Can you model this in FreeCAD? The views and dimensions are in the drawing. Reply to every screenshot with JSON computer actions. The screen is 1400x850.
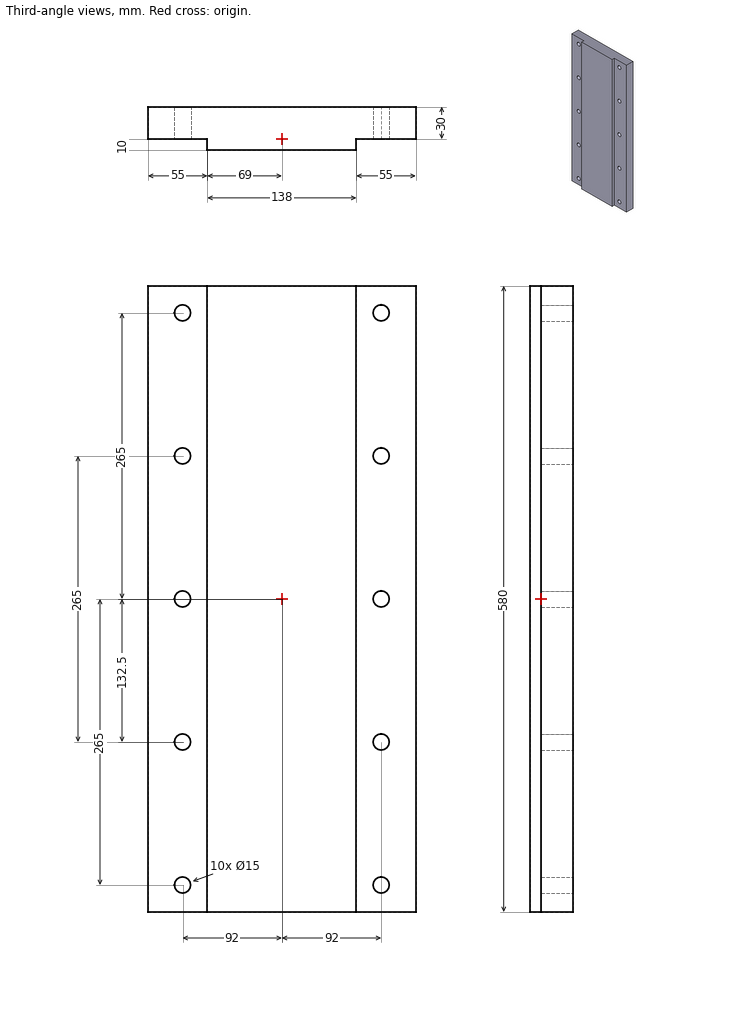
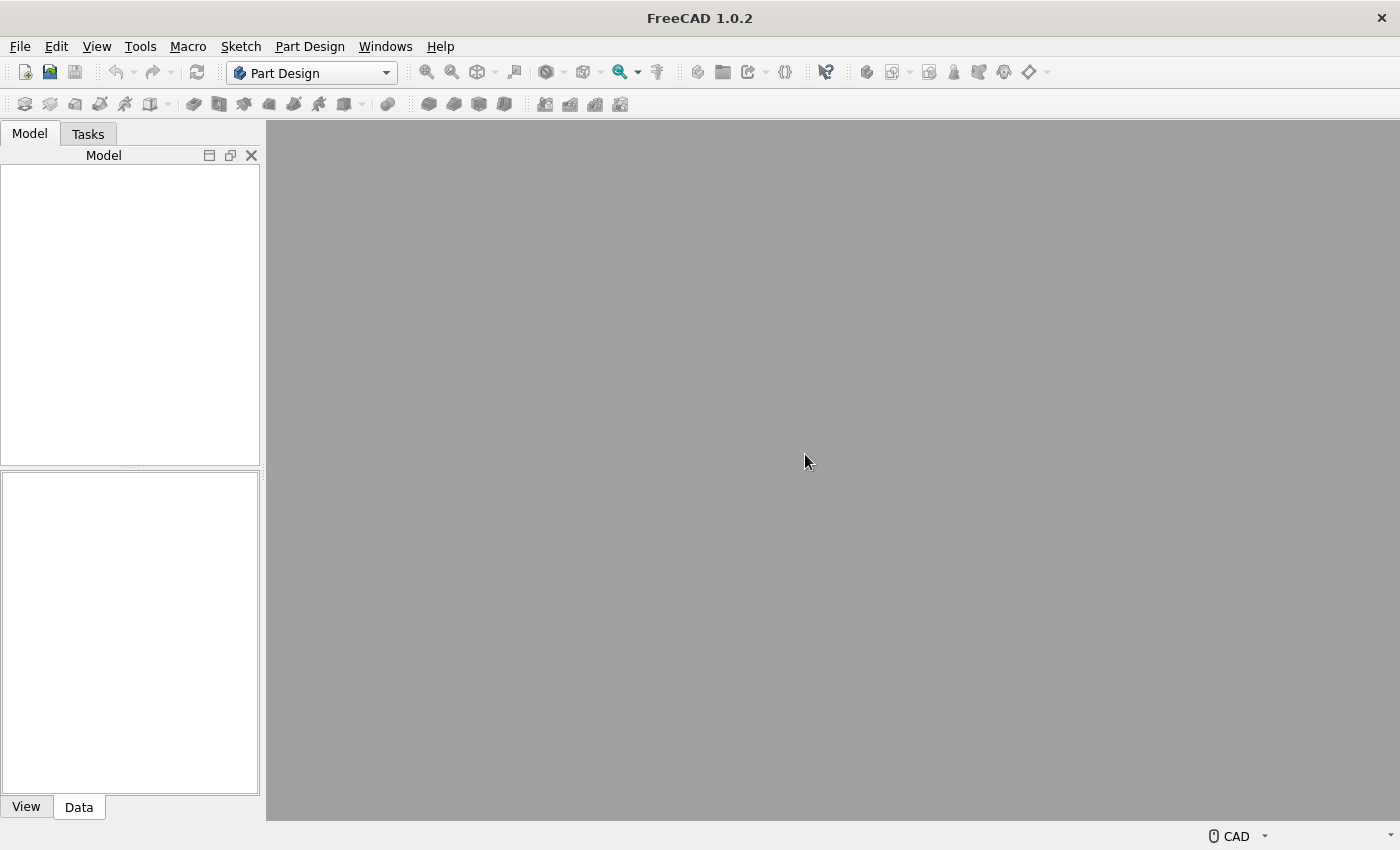
{"action": "left_click", "coordinate": [25, 72]}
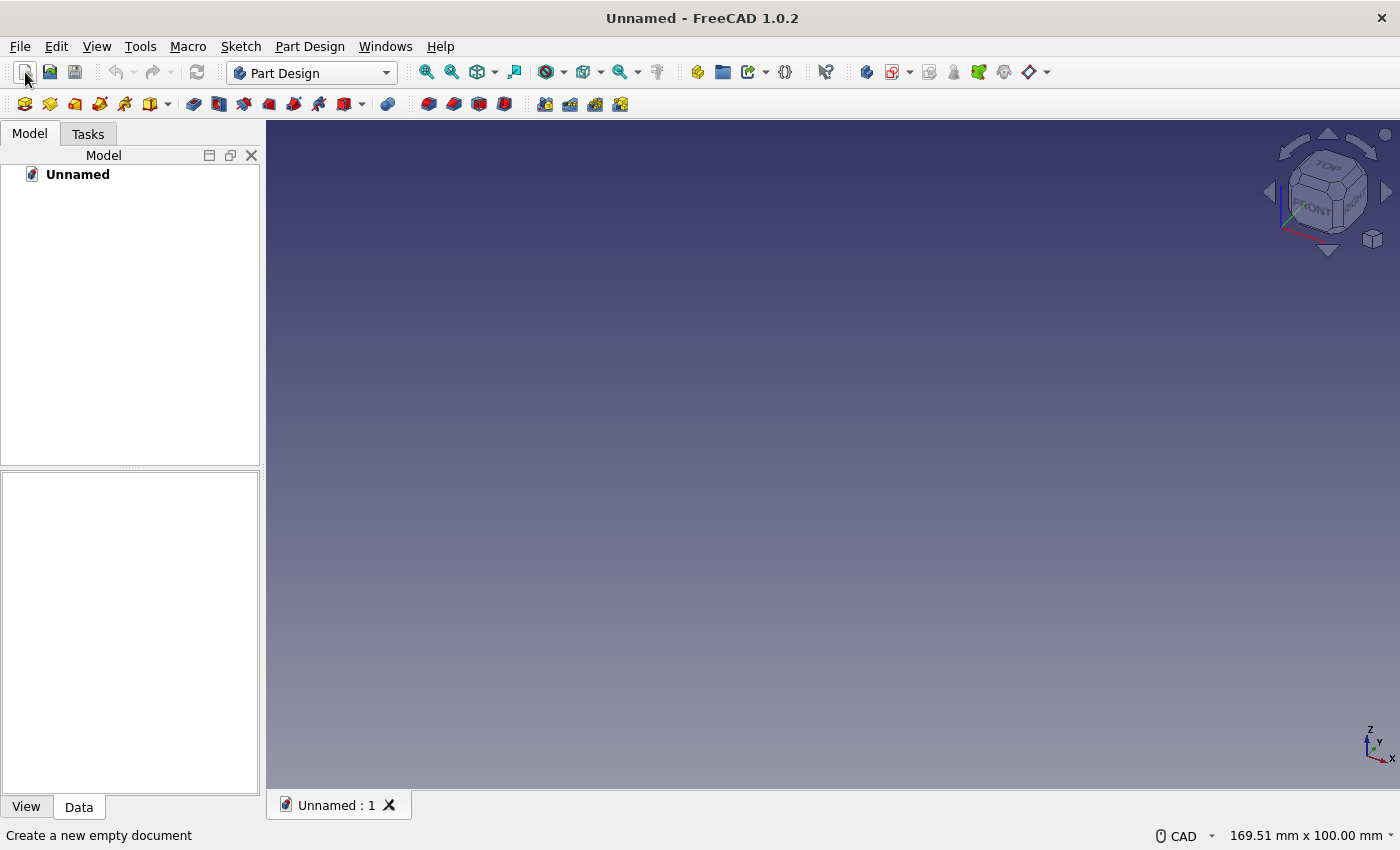
{"action": "left_click", "coordinate": [892, 72]}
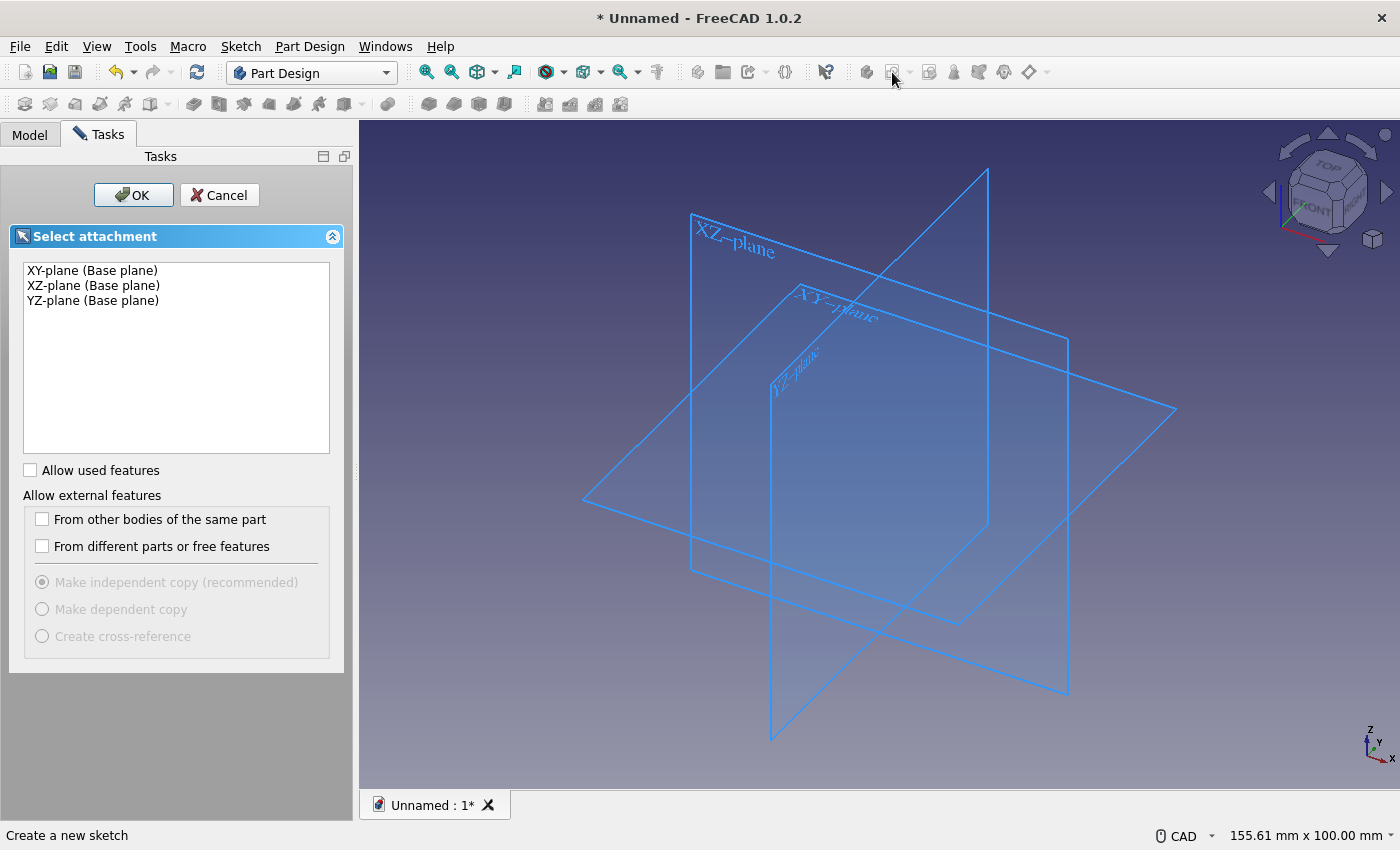
{"action": "left_click", "coordinate": [84, 270]}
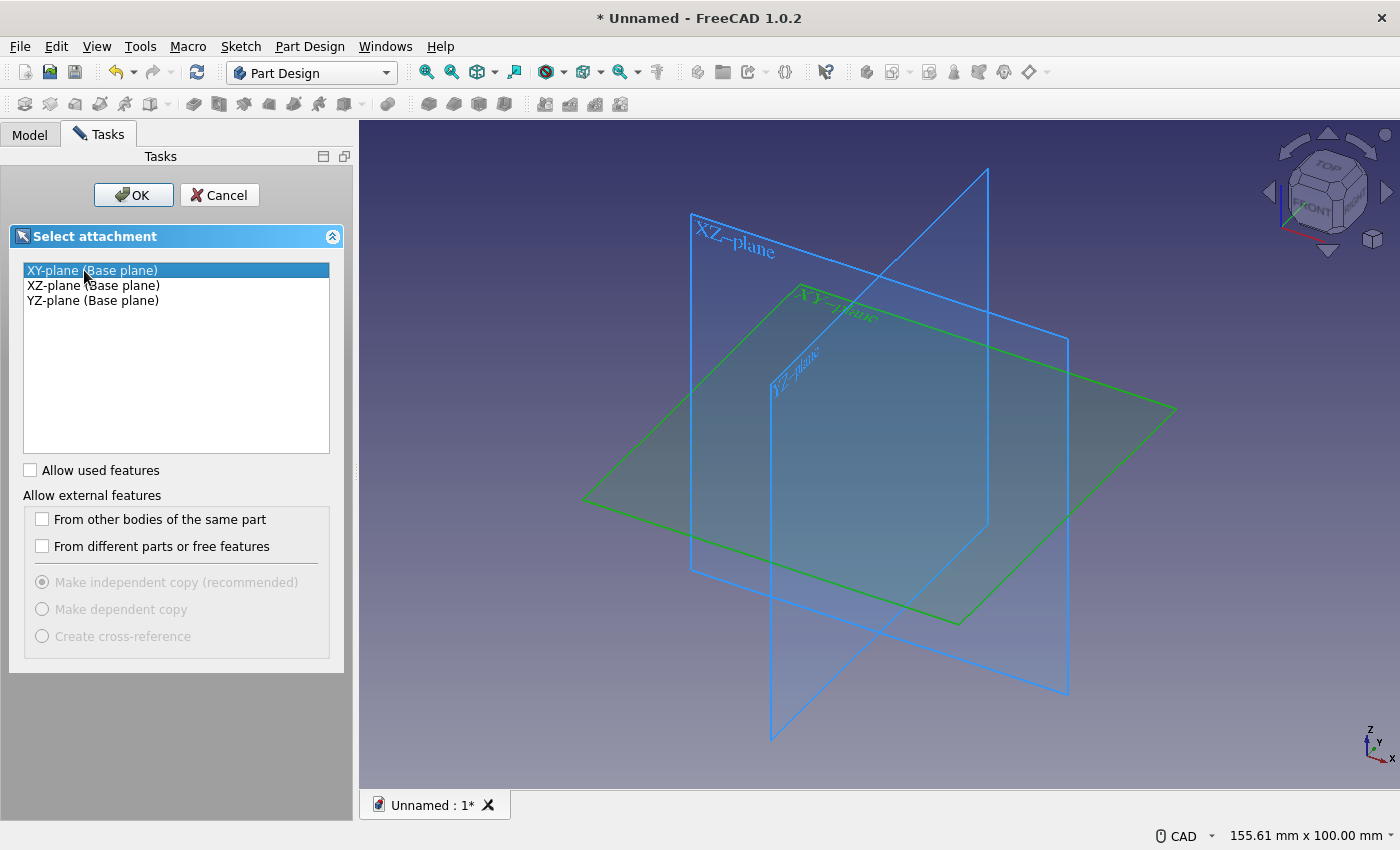
{"action": "left_click", "coordinate": [134, 195]}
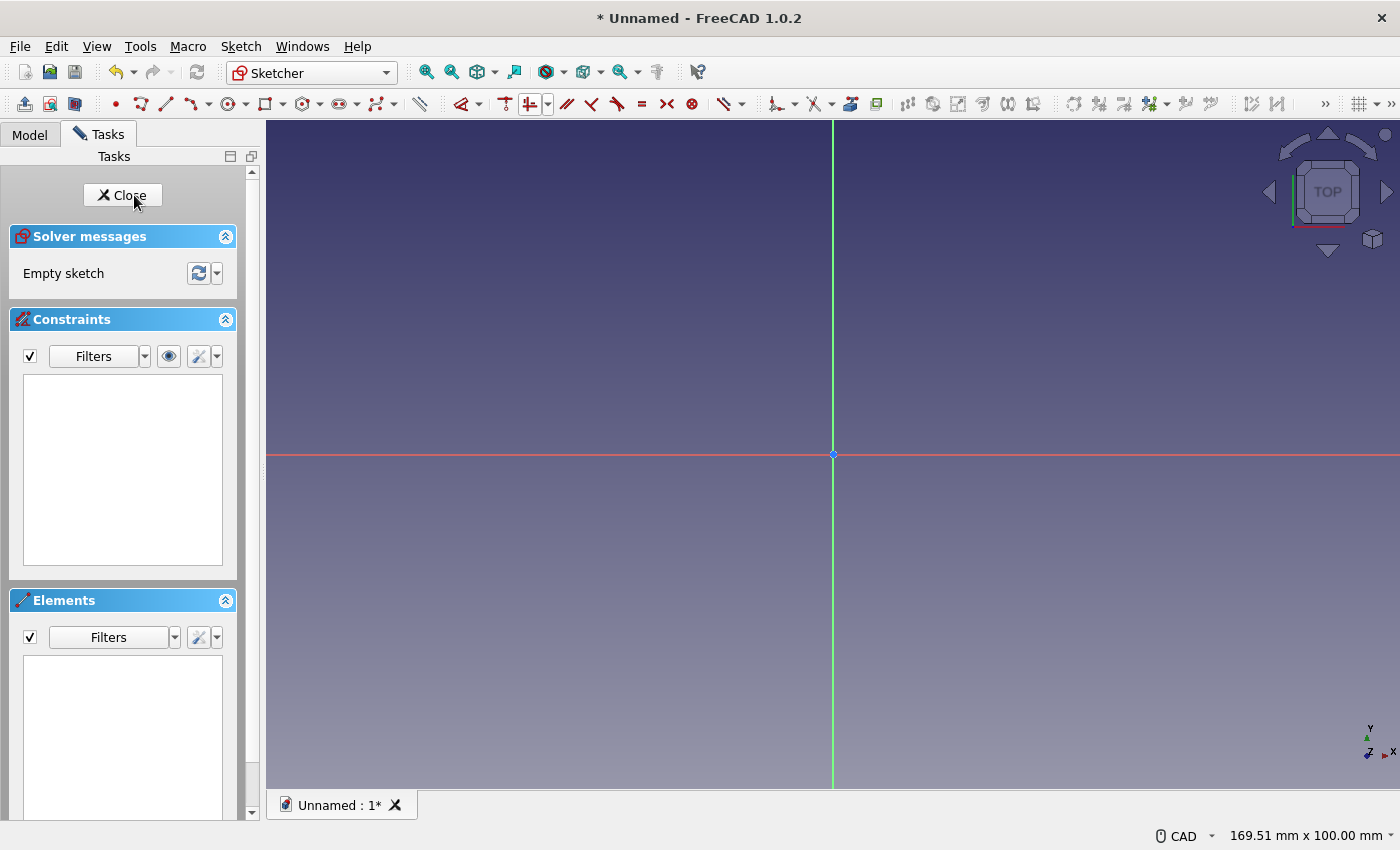
{"action": "scroll", "coordinate": [725, 493], "scroll_direction": "down", "scroll_amount": 5}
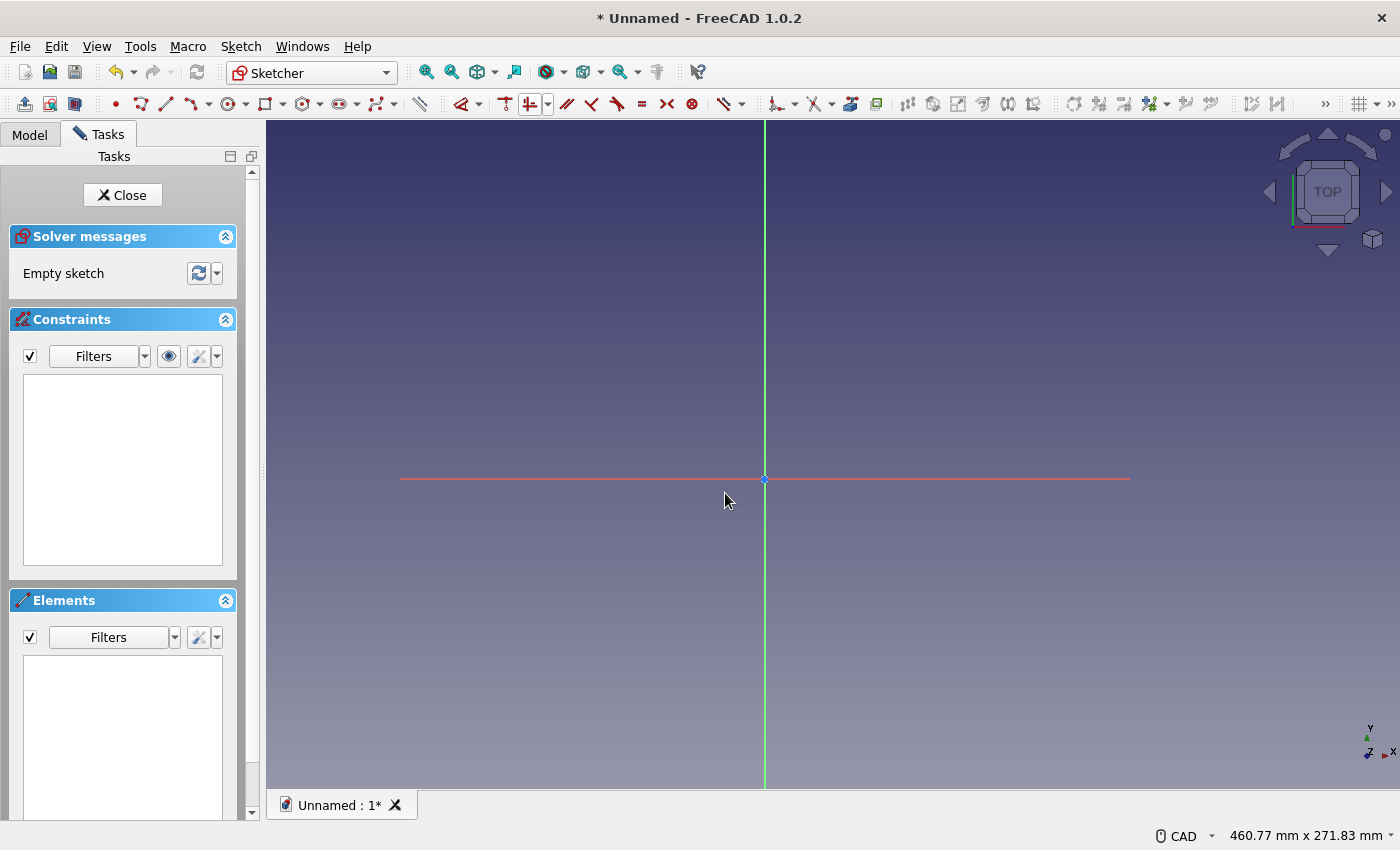
{"action": "key", "text": "g m"}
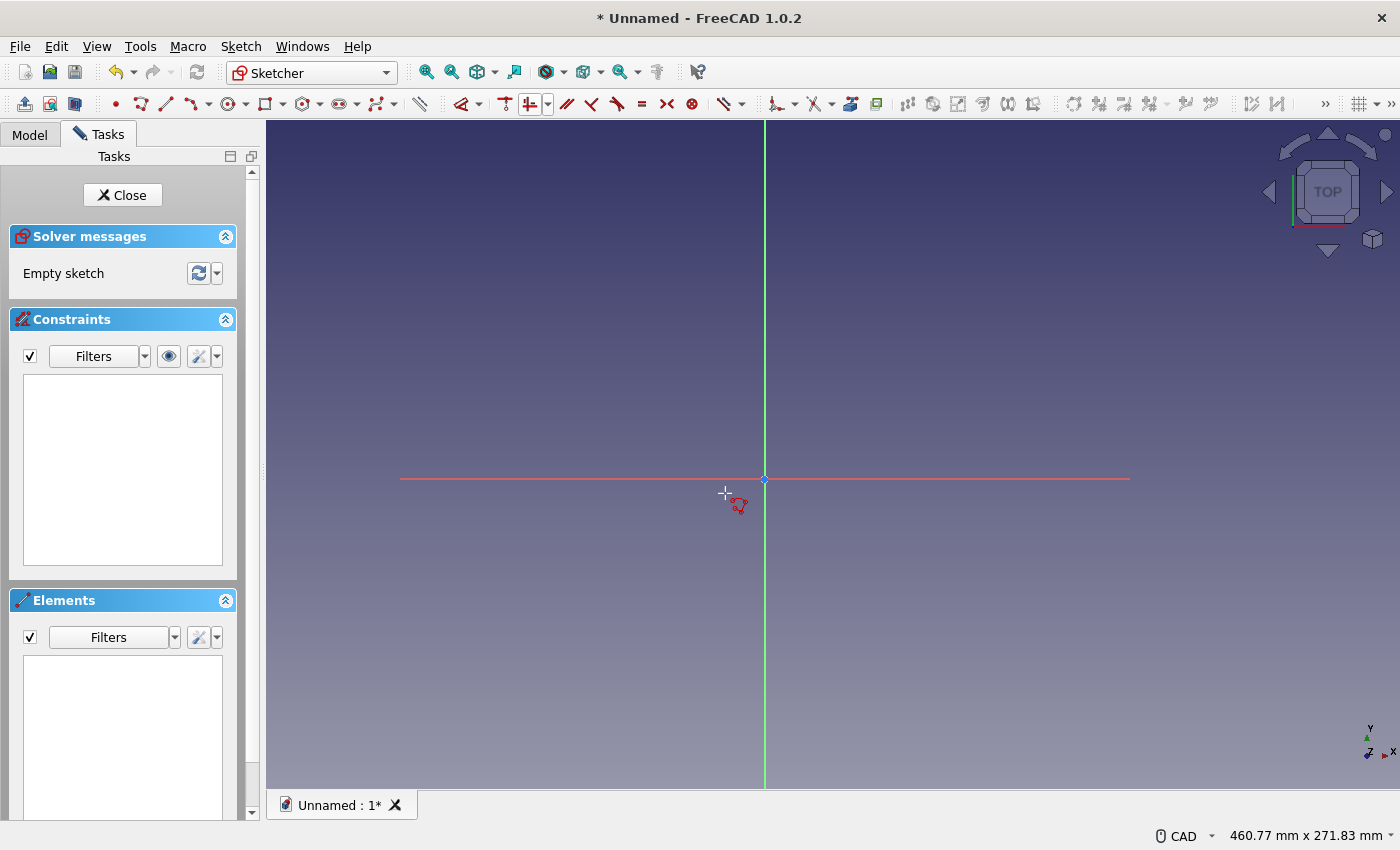
{"action": "left_click", "coordinate": [595, 479]}
{"action": "left_click", "coordinate": [595, 504]}
{"action": "left_click", "coordinate": [935, 504]}
{"action": "left_click", "coordinate": [935, 479]}
{"action": "left_click", "coordinate": [1070, 470]}
{"action": "left_click", "coordinate": [1070, 405]}
{"action": "left_click", "coordinate": [460, 405]}
{"action": "left_click", "coordinate": [460, 470]}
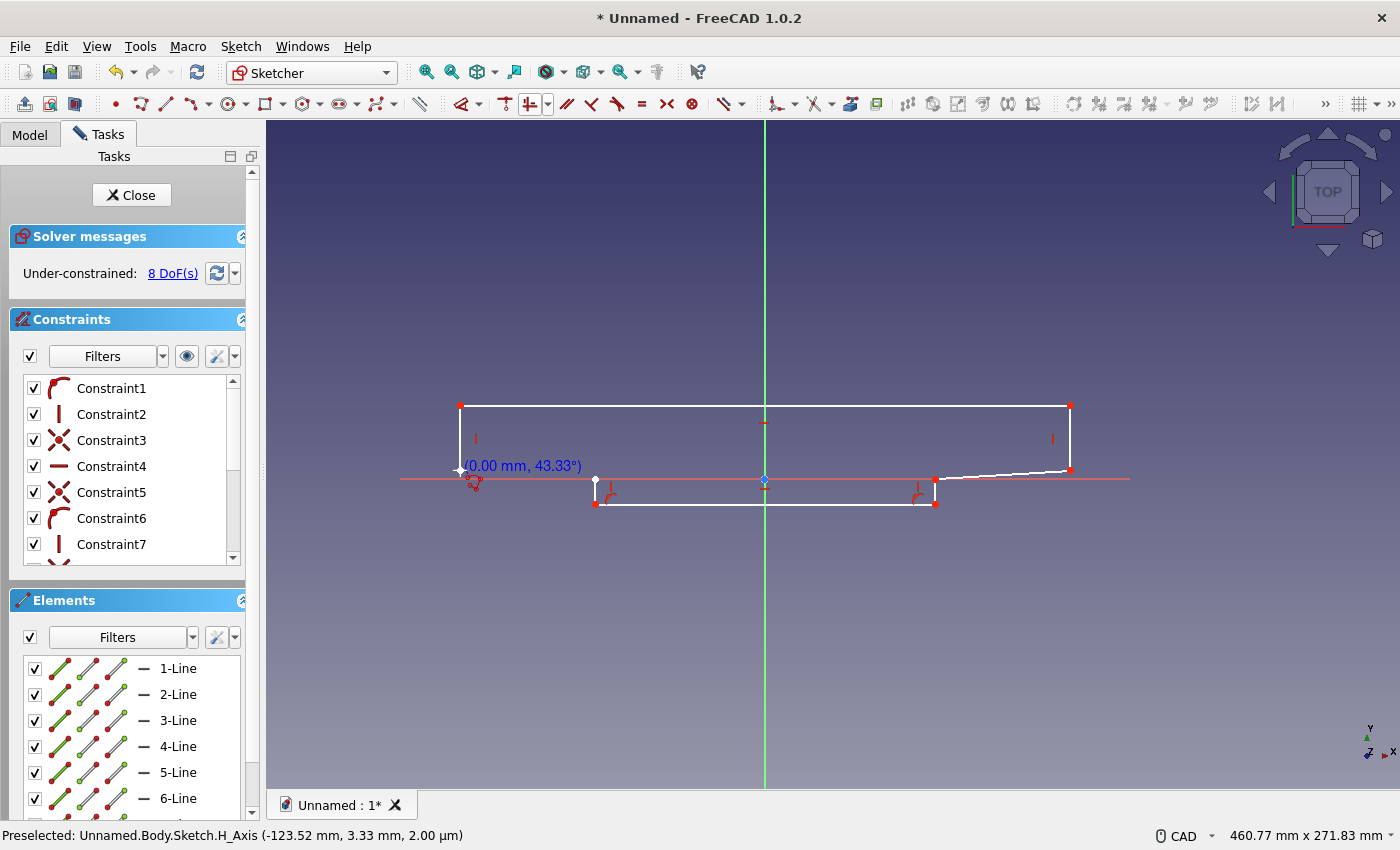
{"action": "scroll", "coordinate": [595, 479], "scroll_direction": "up", "scroll_amount": 2}